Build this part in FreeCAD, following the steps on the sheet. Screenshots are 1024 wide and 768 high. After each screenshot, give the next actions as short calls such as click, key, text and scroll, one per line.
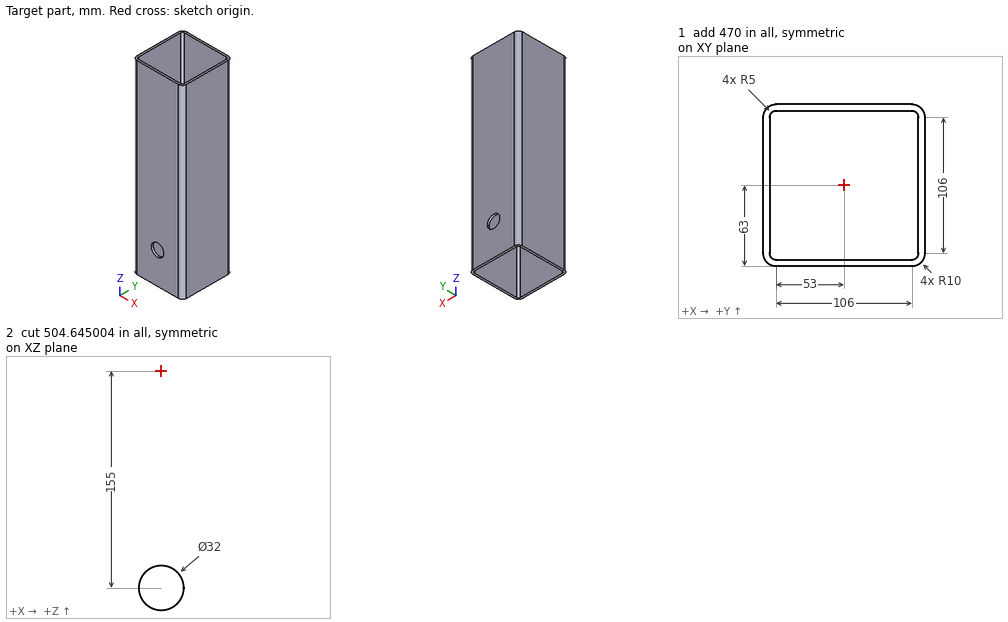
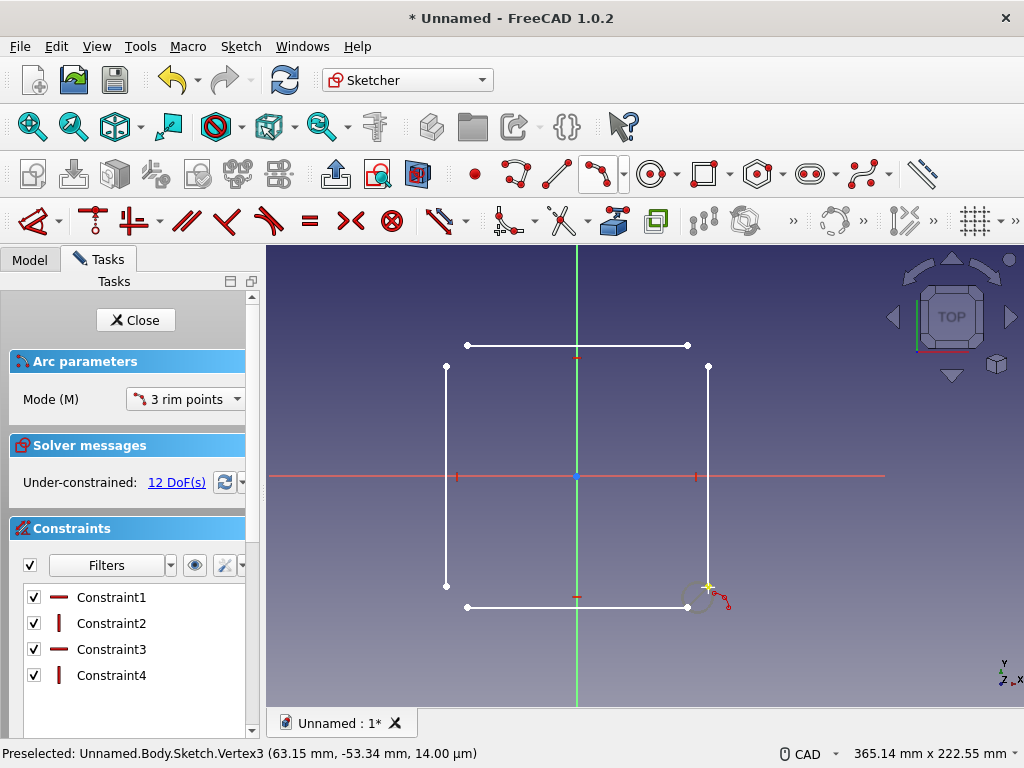
scroll(702, 601, up, 5)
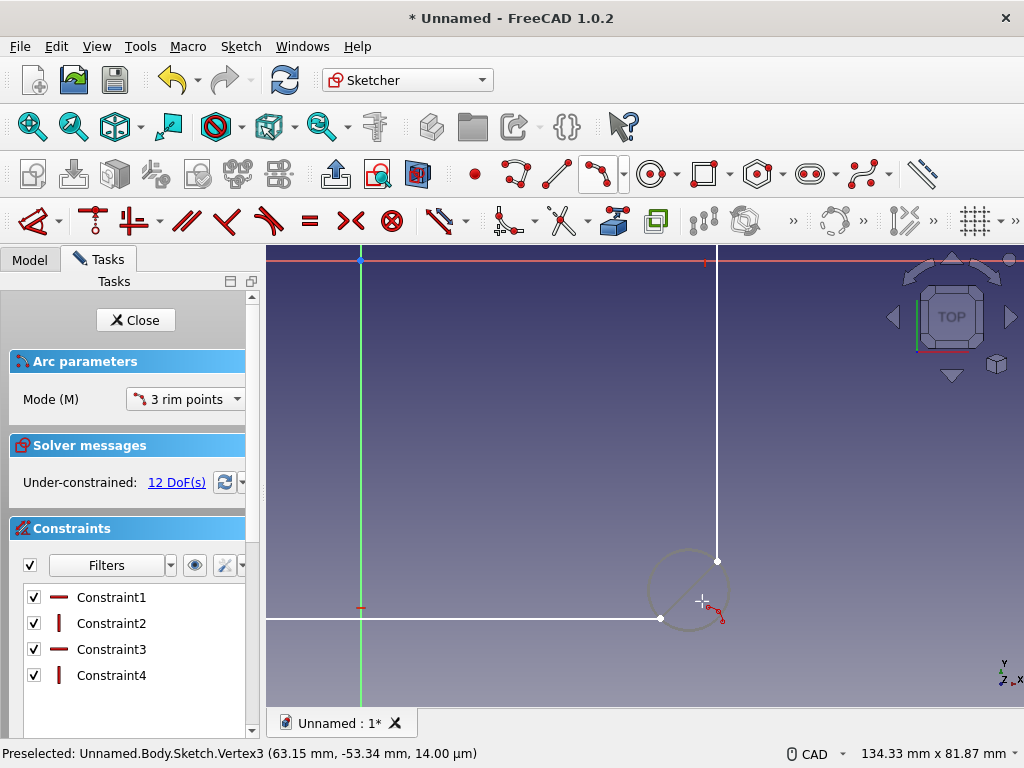
click(700, 600)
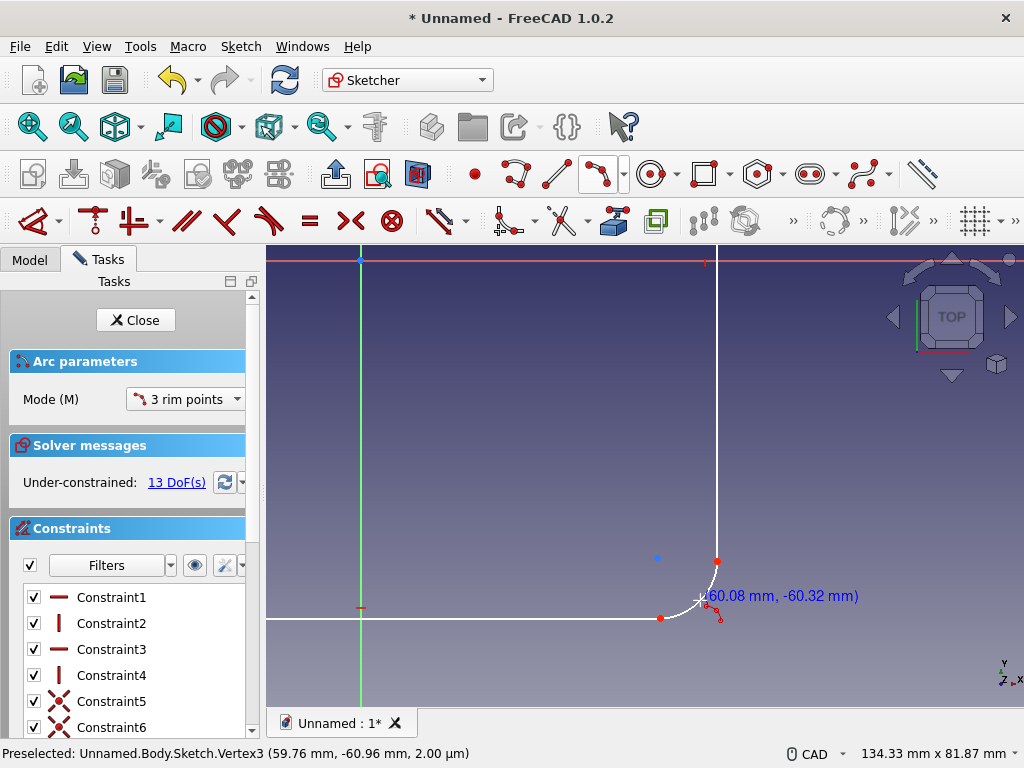
scroll(702, 601, down, 5)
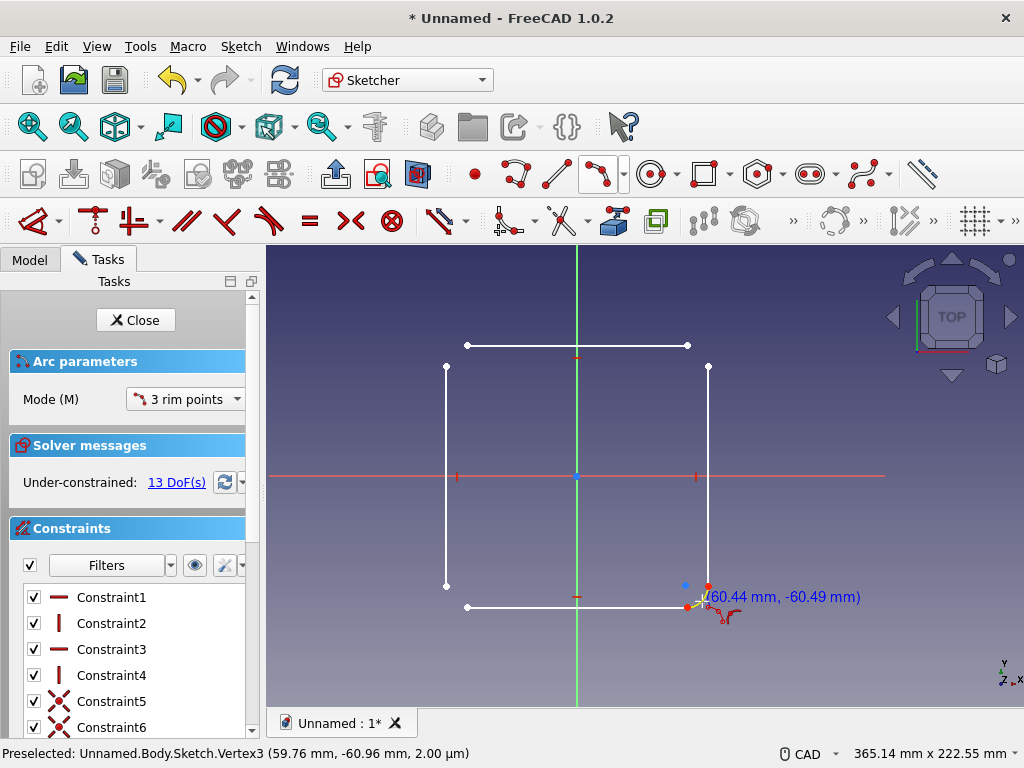
click(708, 367)
click(687, 346)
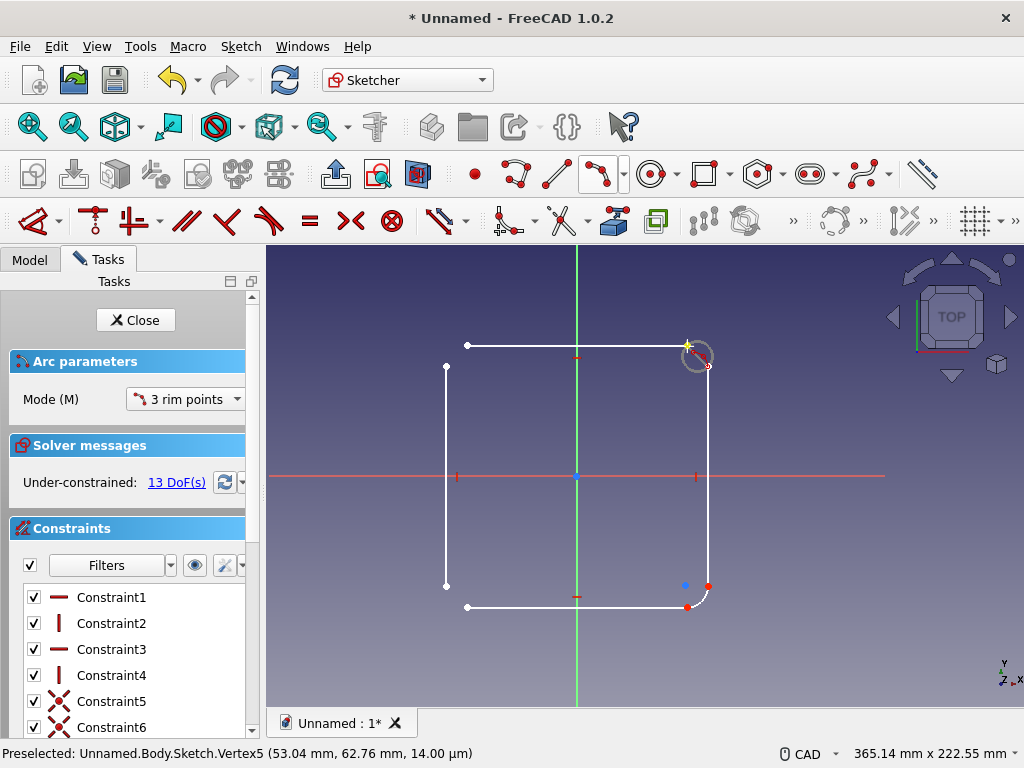
scroll(702, 352, up, 5)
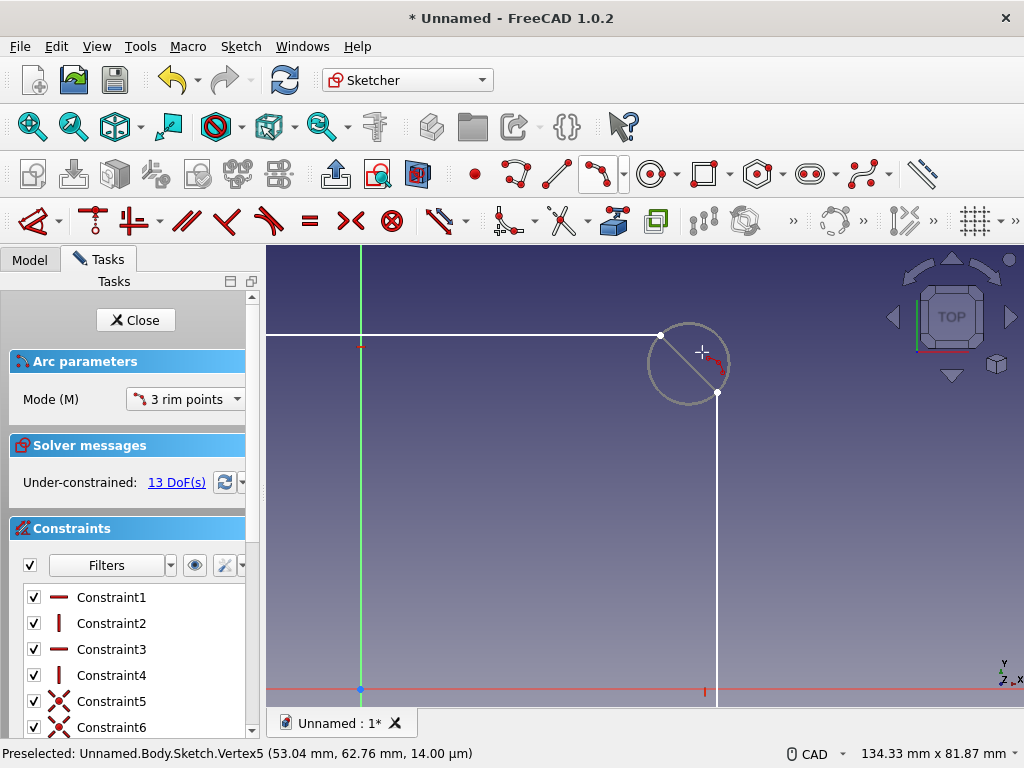
click(700, 350)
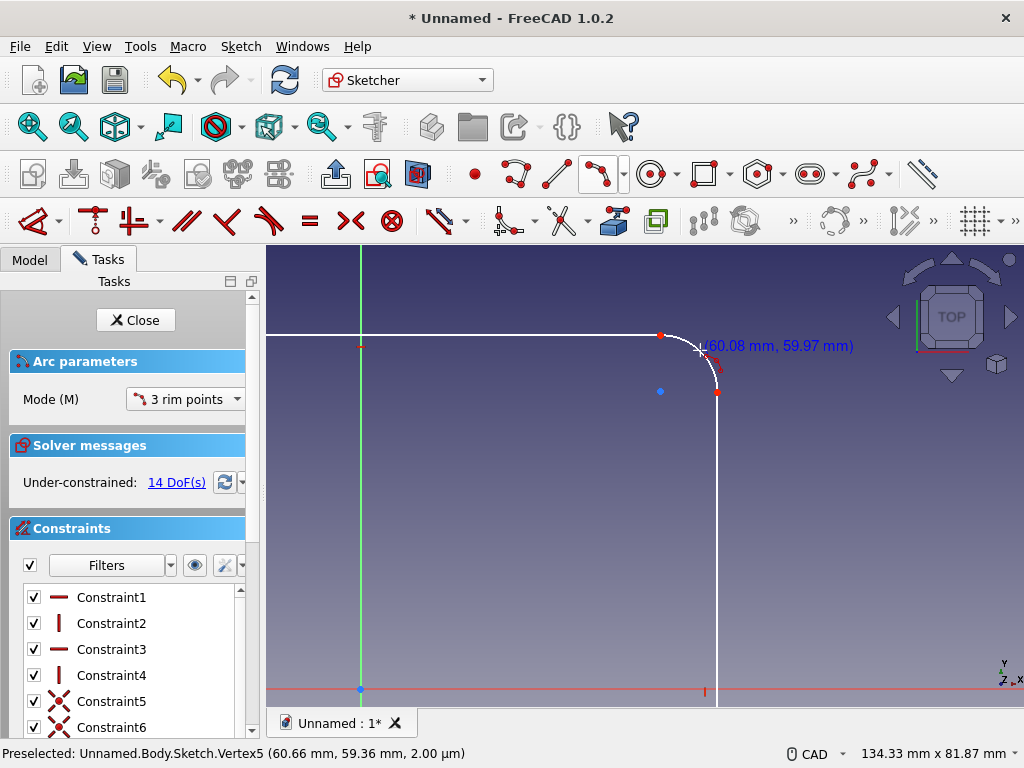
scroll(702, 352, down, 5)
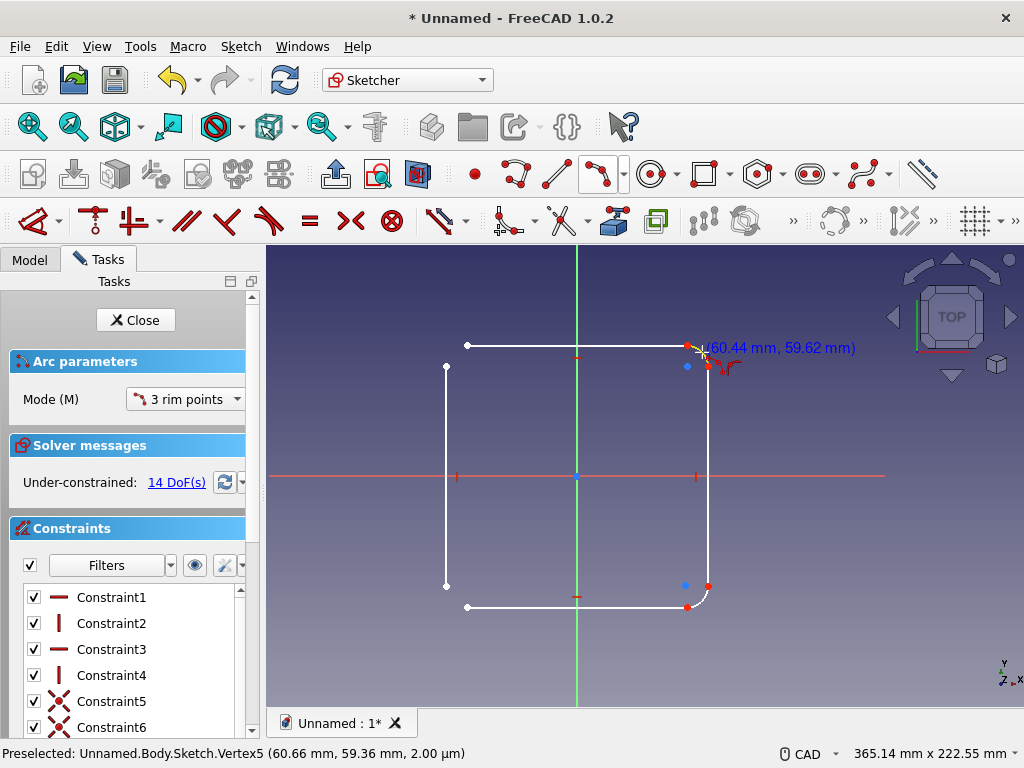
click(467, 346)
click(446, 367)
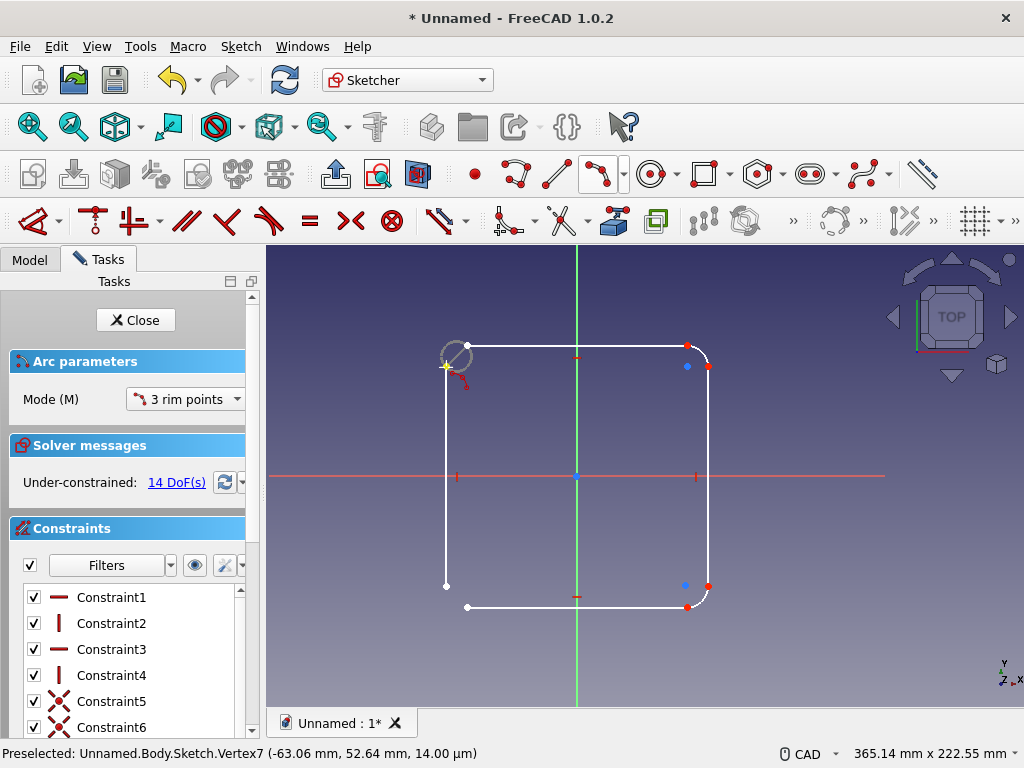
scroll(452, 352, up, 5)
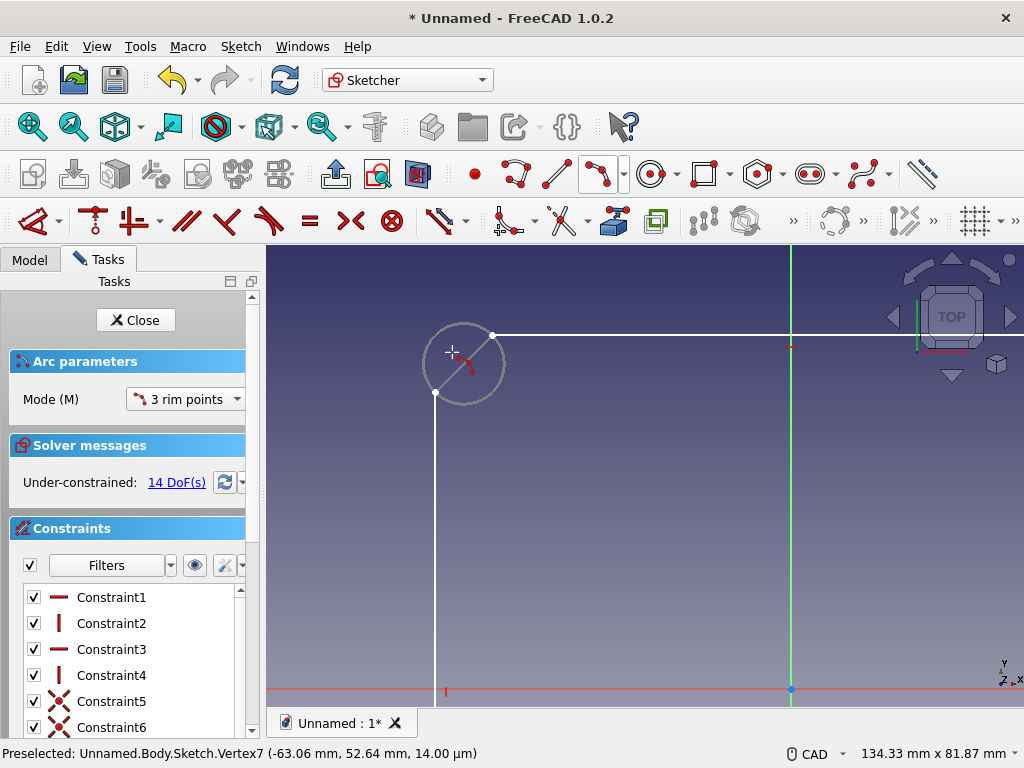
click(452, 350)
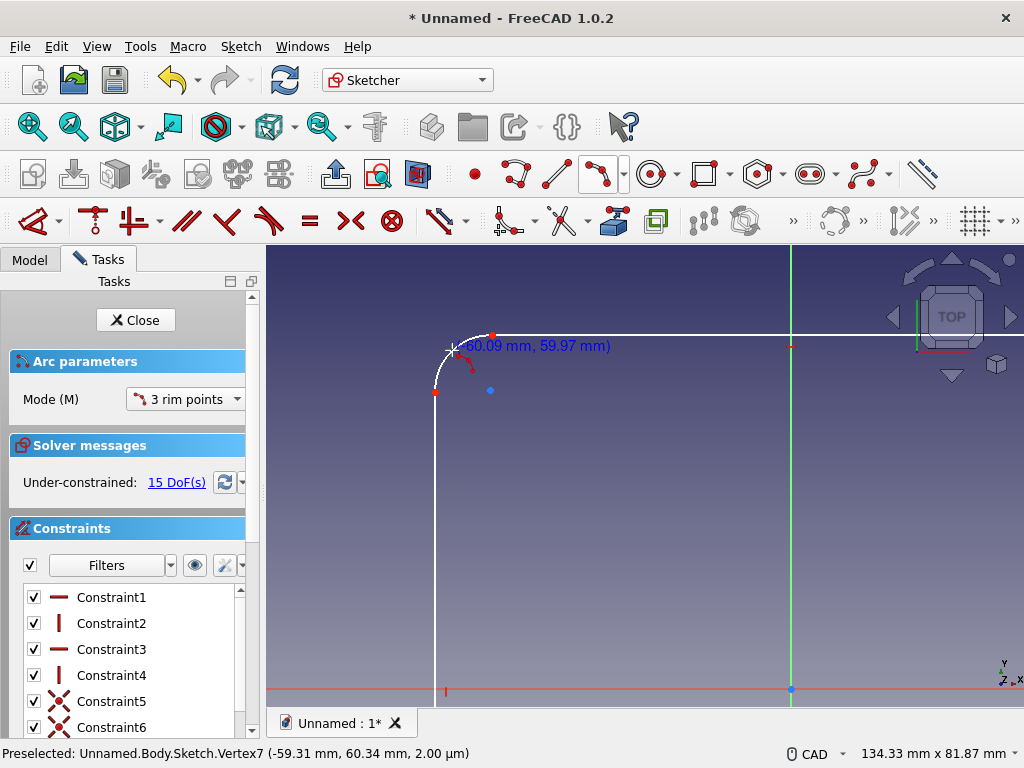
scroll(452, 352, down, 5)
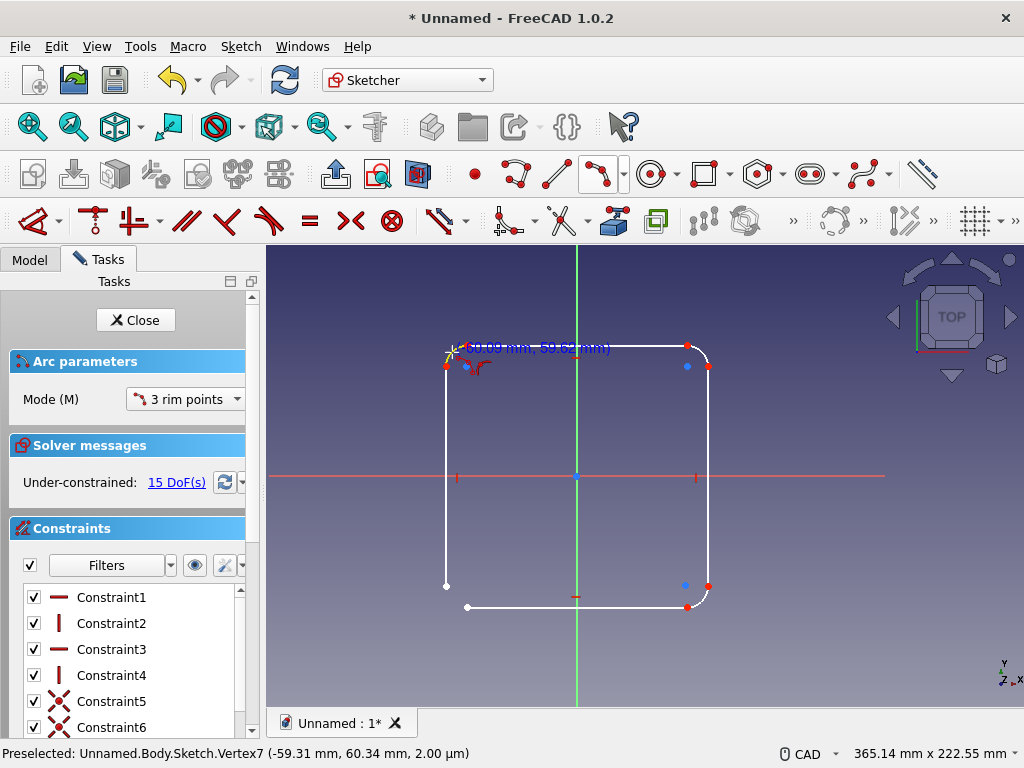
click(446, 587)
click(467, 608)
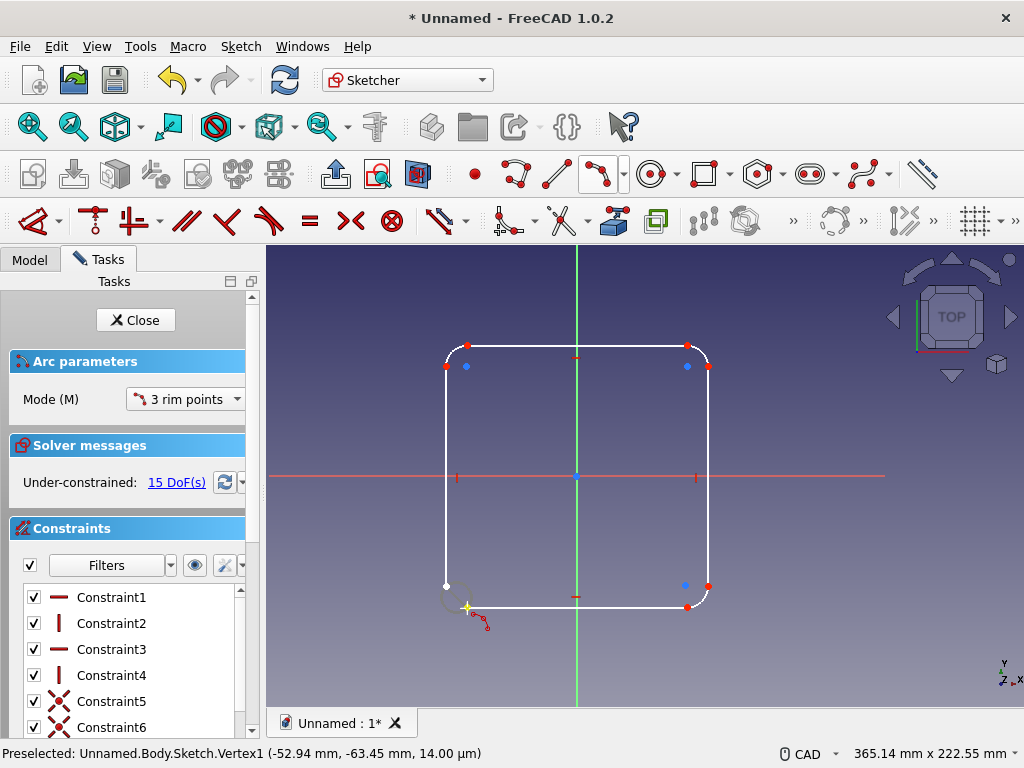
scroll(452, 601, up, 5)